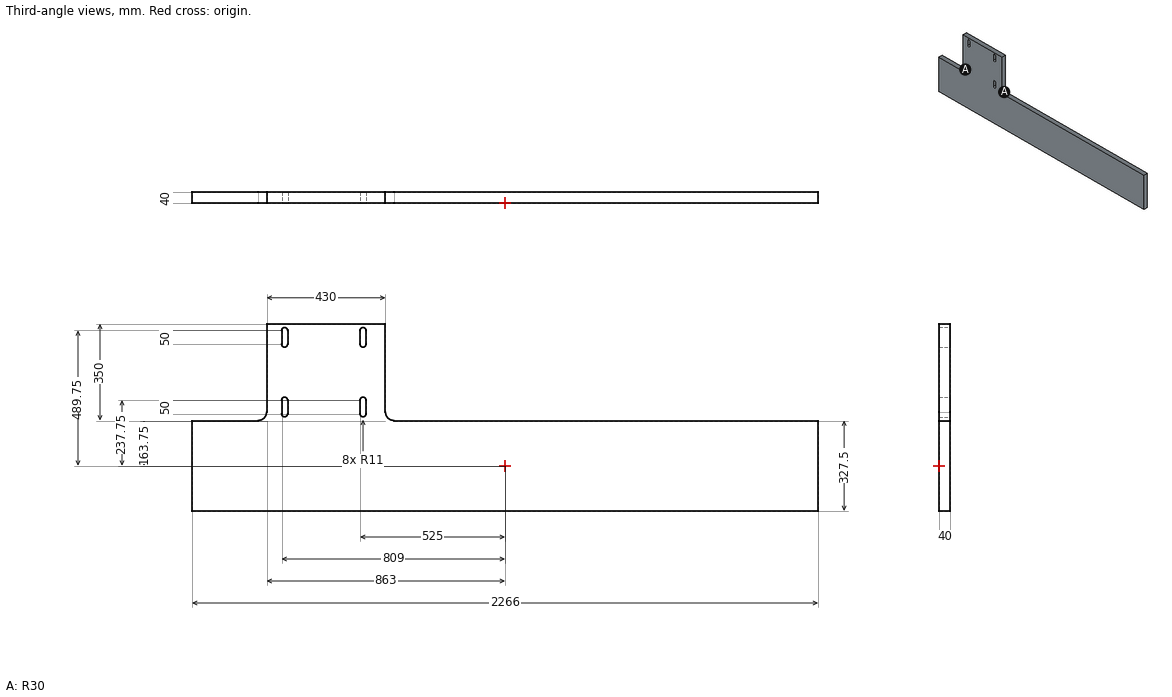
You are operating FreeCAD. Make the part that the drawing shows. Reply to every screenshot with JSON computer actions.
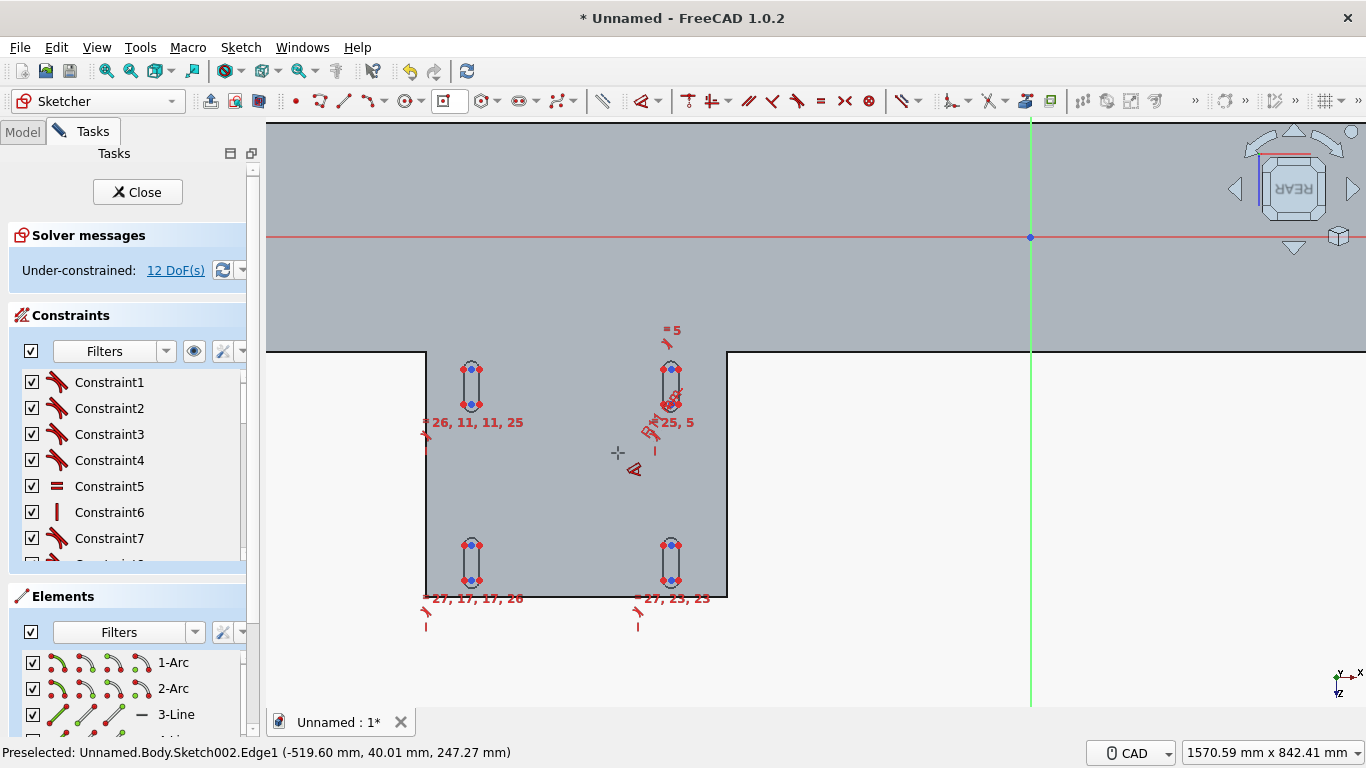
{"action": "scroll", "coordinate": [663, 394], "scroll_direction": "up", "scroll_amount": 2}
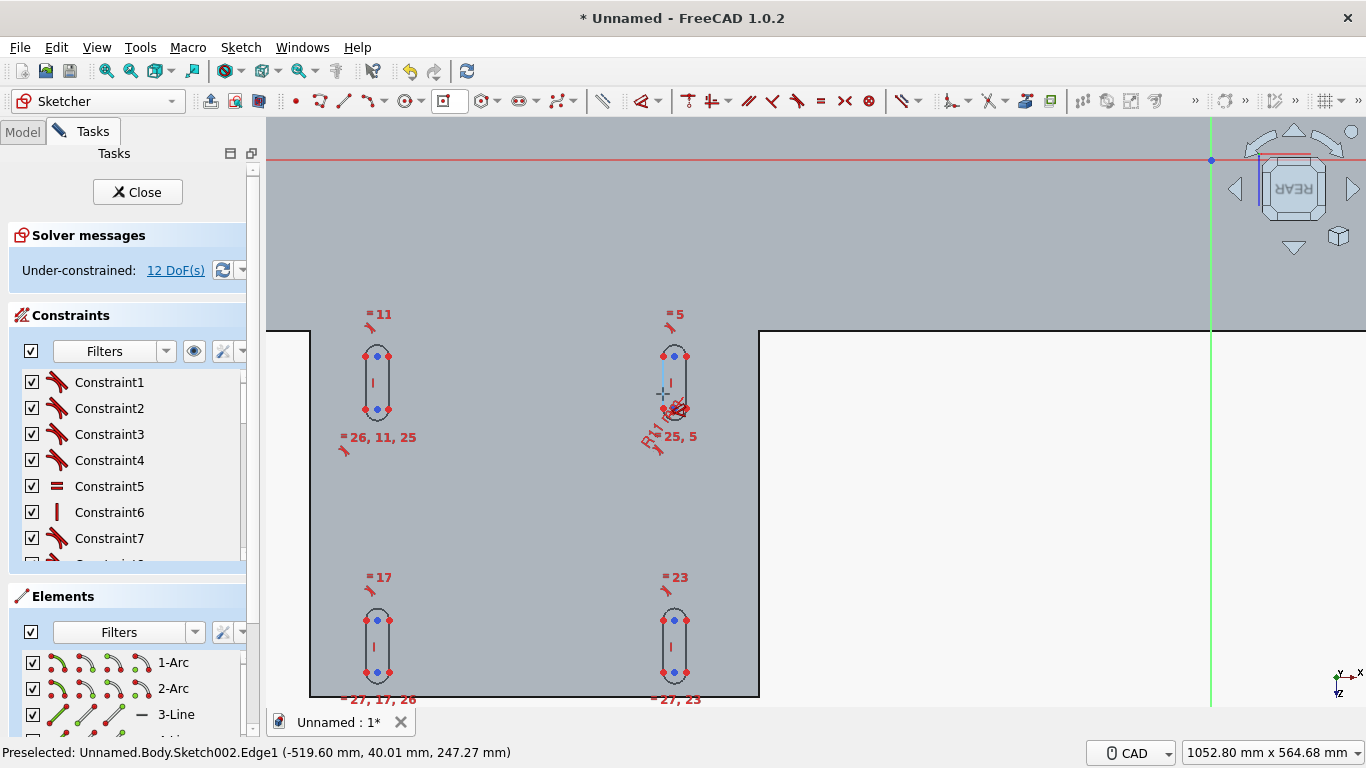
{"action": "left_click", "coordinate": [663, 393]}
{"action": "left_click", "coordinate": [629, 383]}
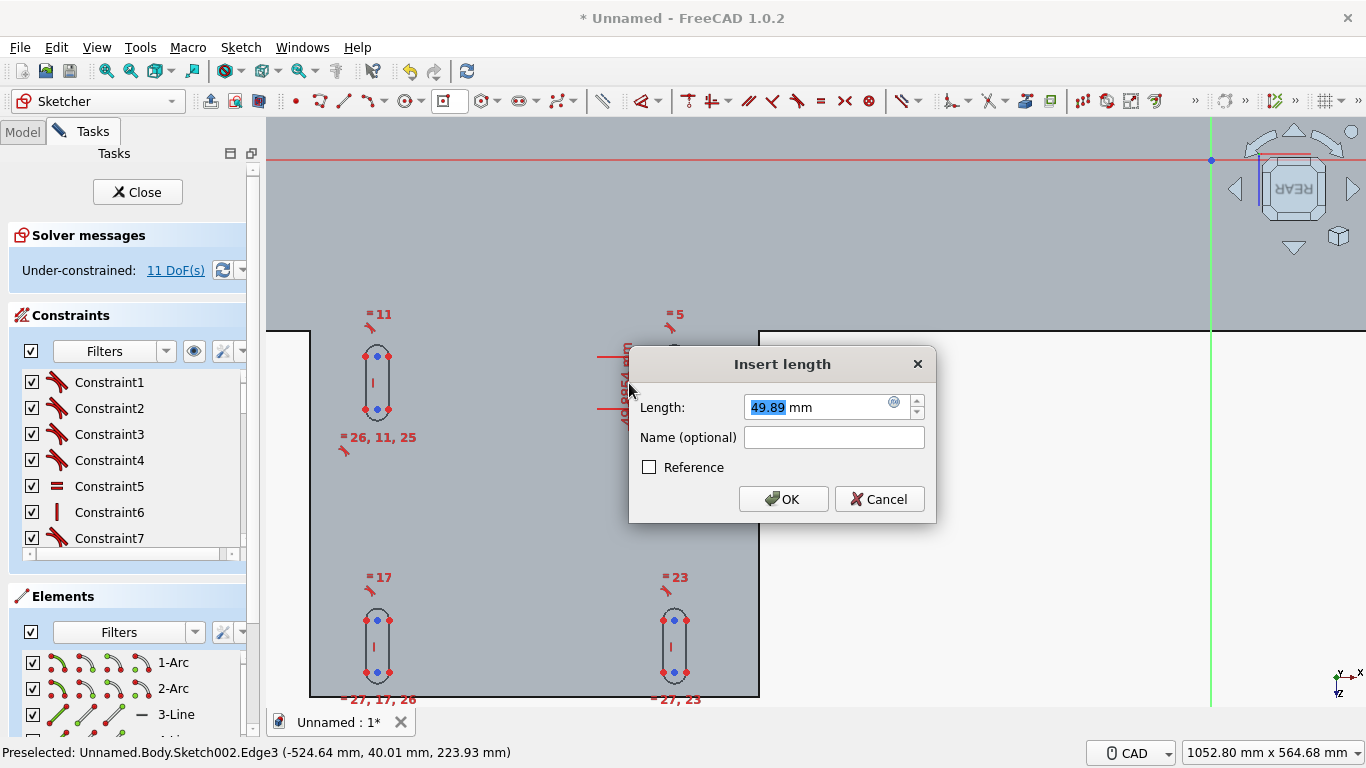
{"action": "type", "text": "50"}
{"action": "key", "text": "Return"}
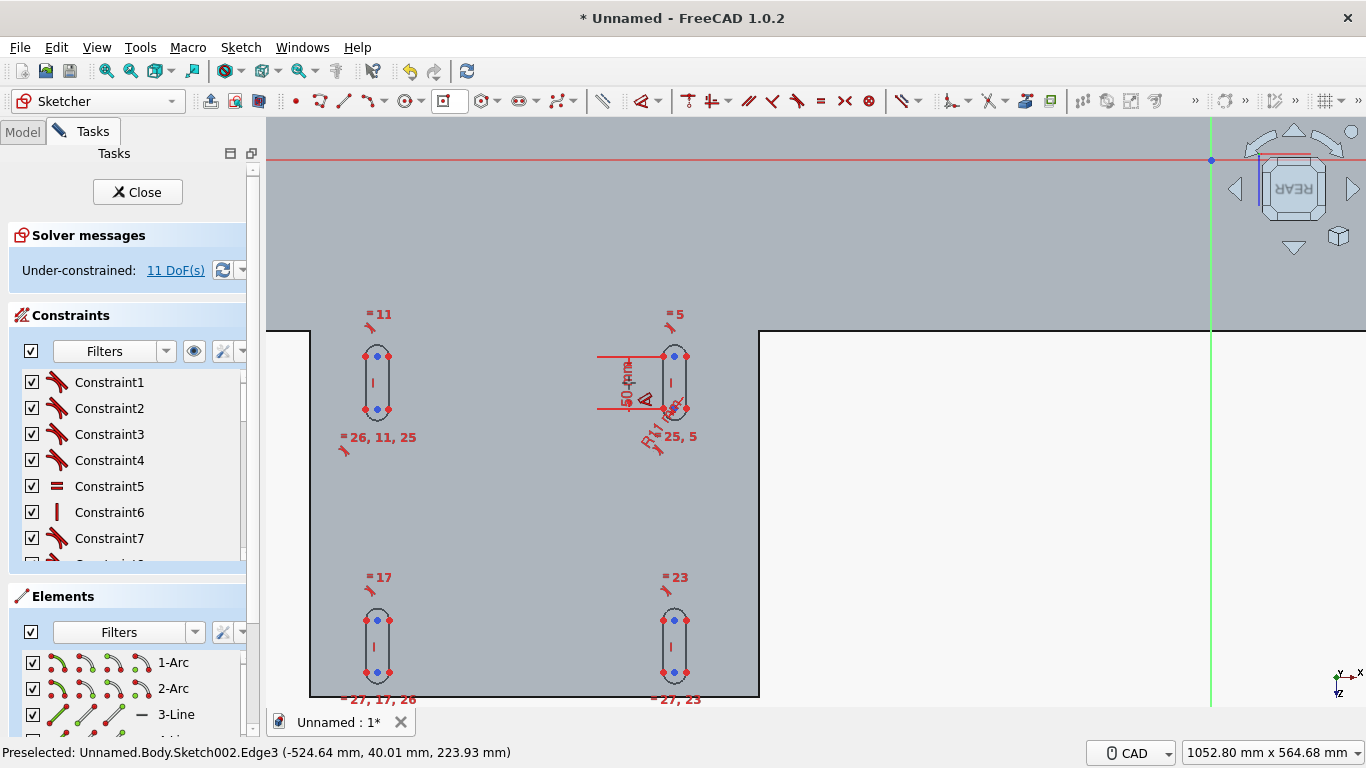
{"action": "left_click", "coordinate": [366, 393]}
{"action": "left_click", "coordinate": [332, 383]}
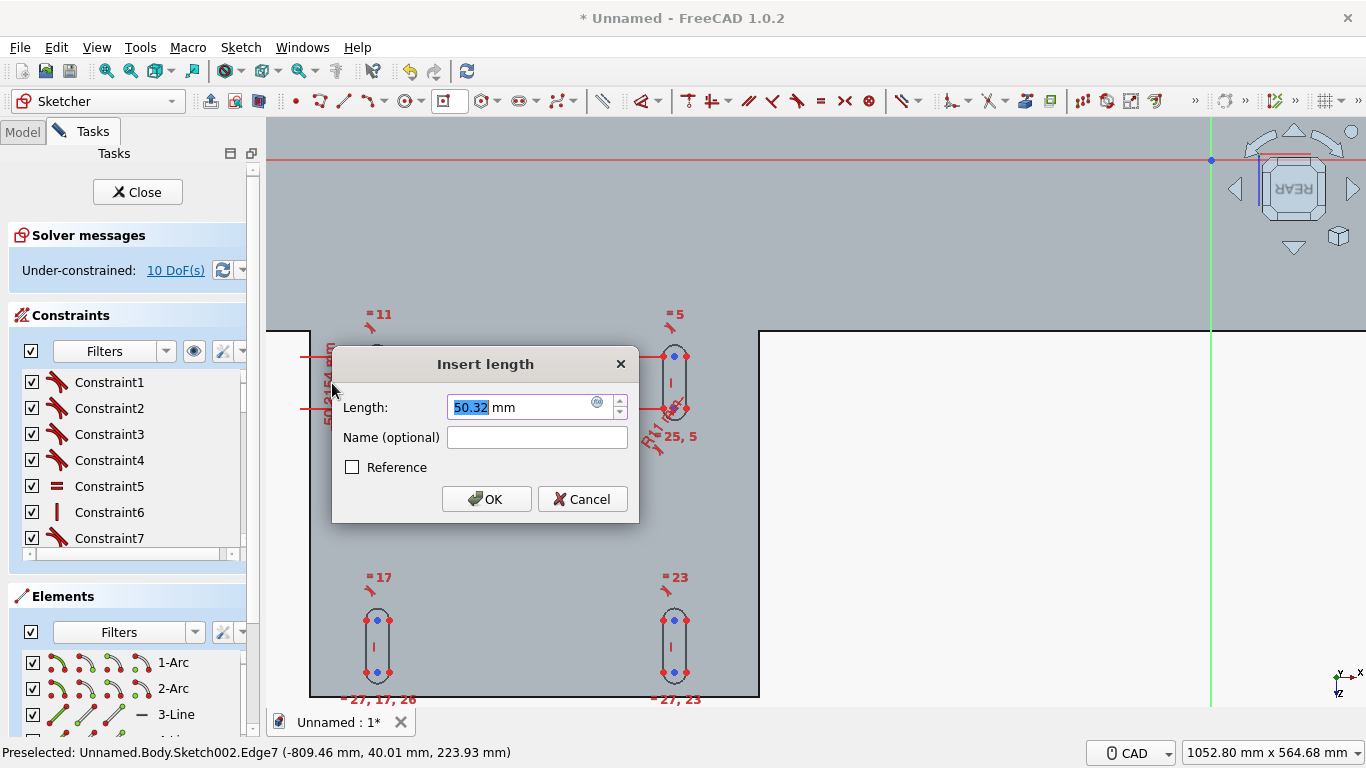
{"action": "type", "text": "50"}
{"action": "key", "text": "Return"}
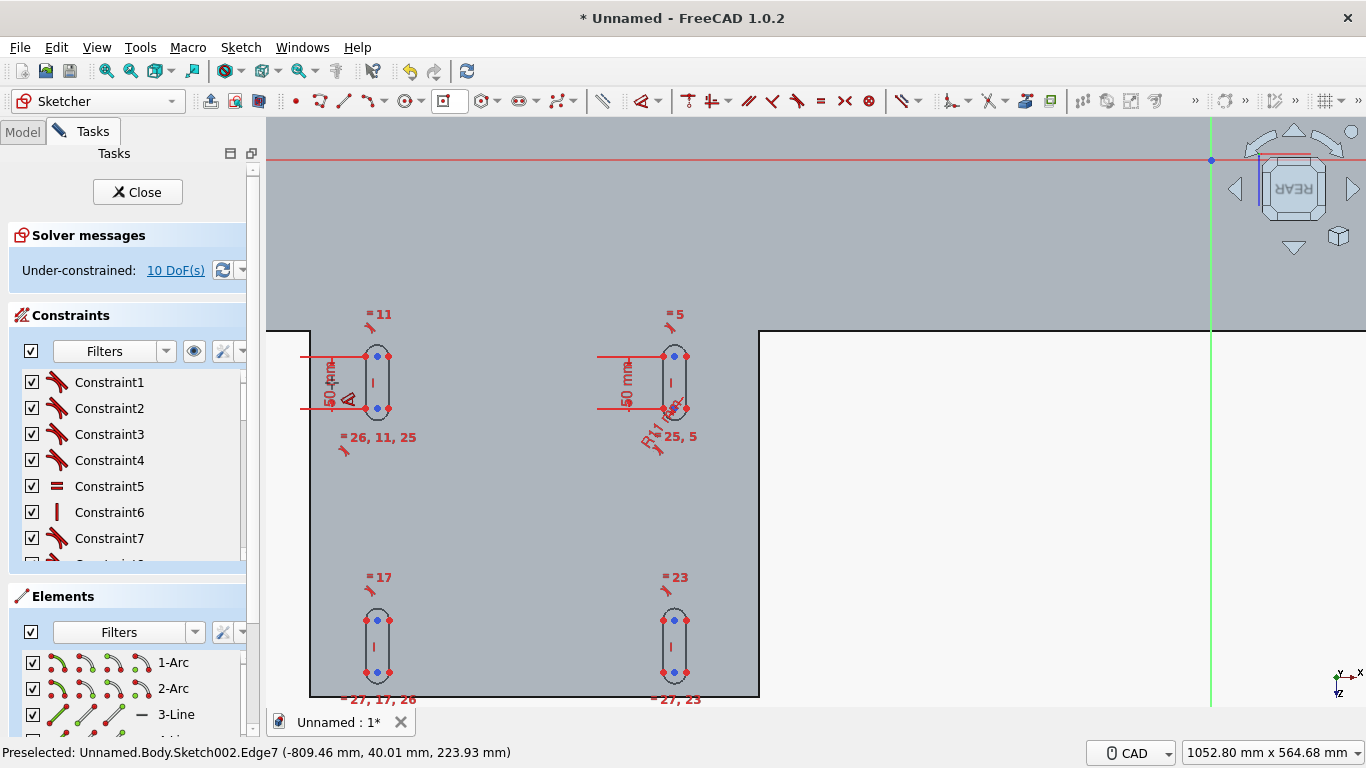
{"action": "left_click", "coordinate": [366, 656]}
{"action": "left_click", "coordinate": [332, 646]}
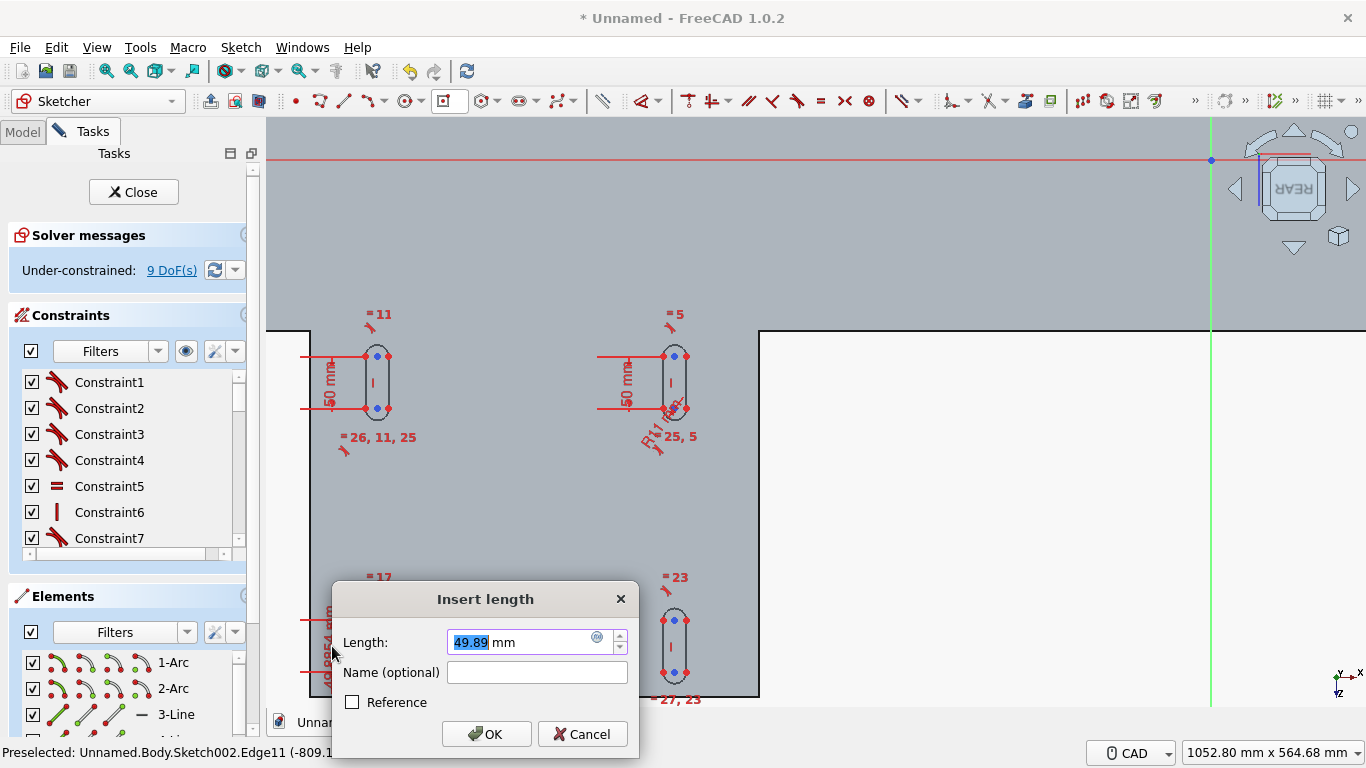
{"action": "type", "text": "50"}
{"action": "key", "text": "Return"}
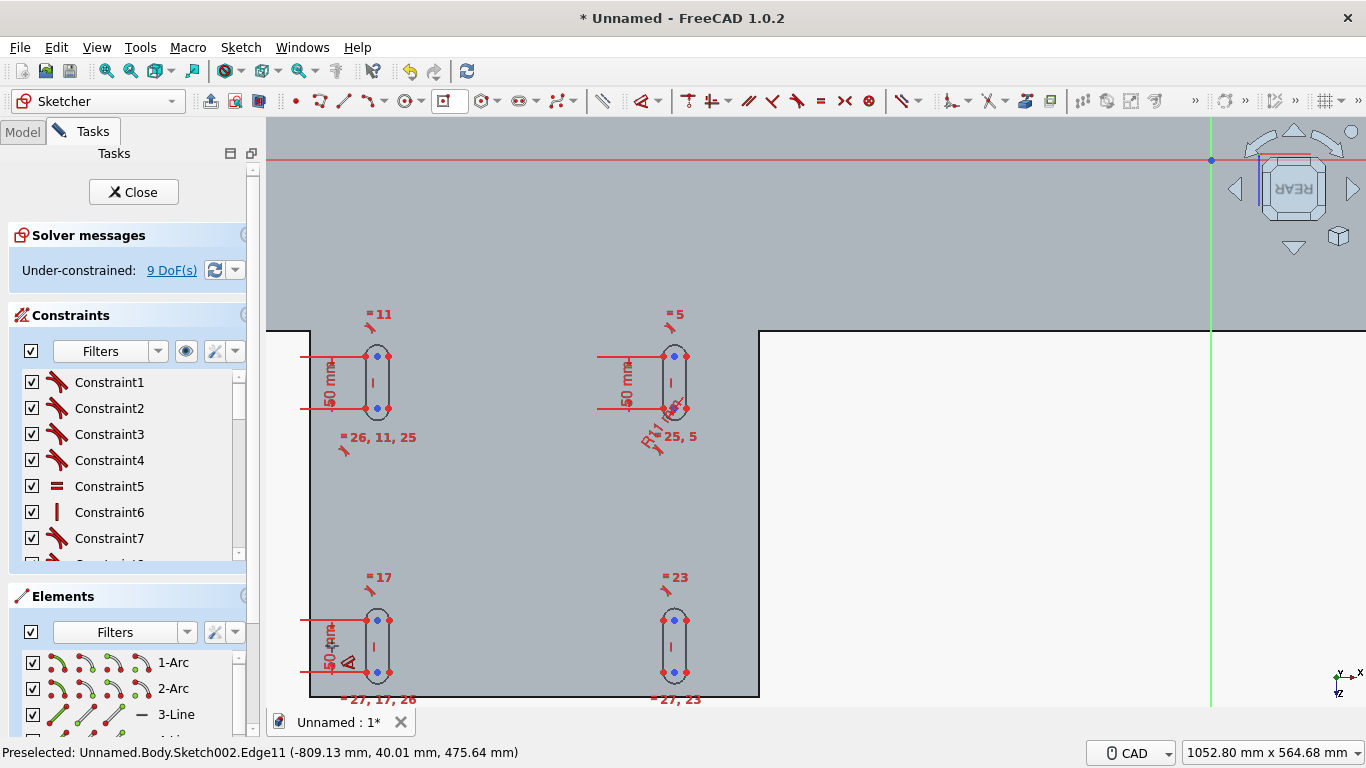
{"action": "left_click", "coordinate": [663, 656]}
{"action": "left_click", "coordinate": [629, 646]}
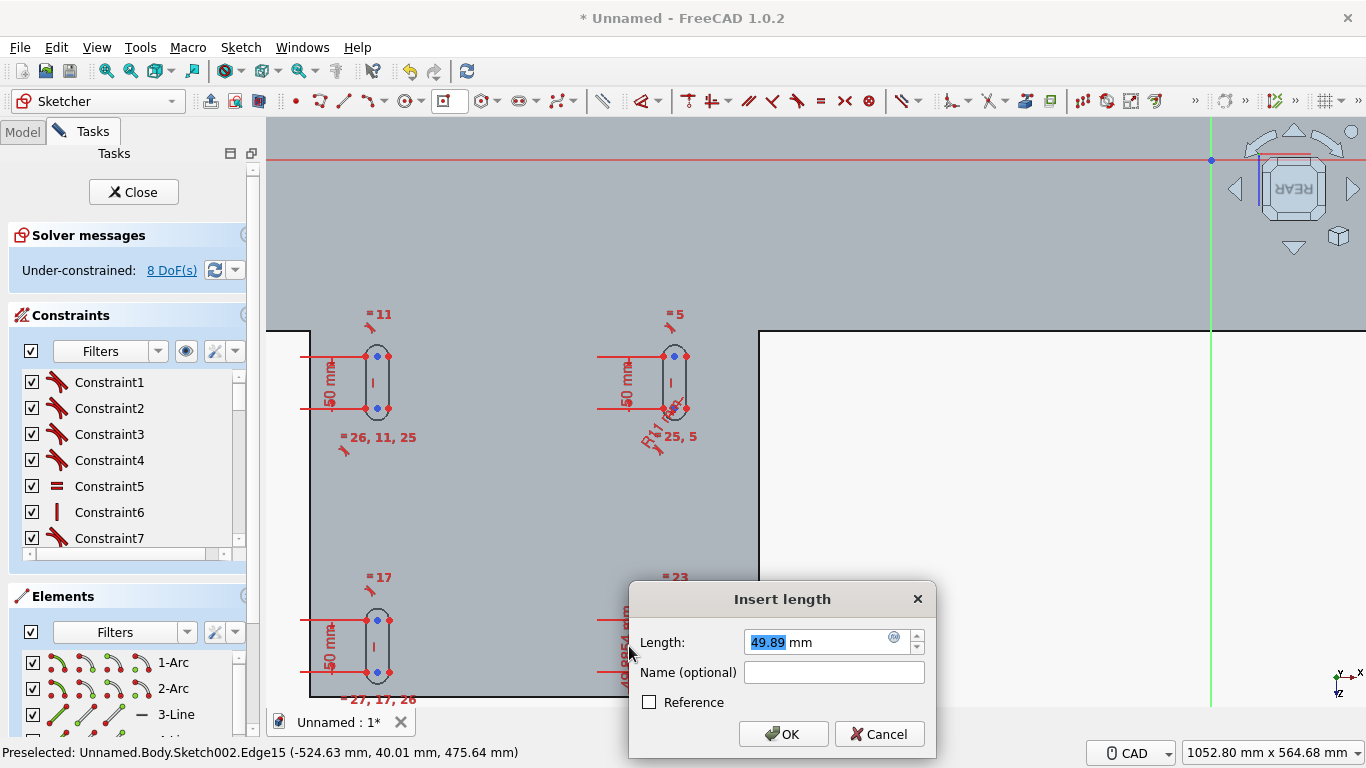
{"action": "type", "text": "50"}
{"action": "key", "text": "Return"}